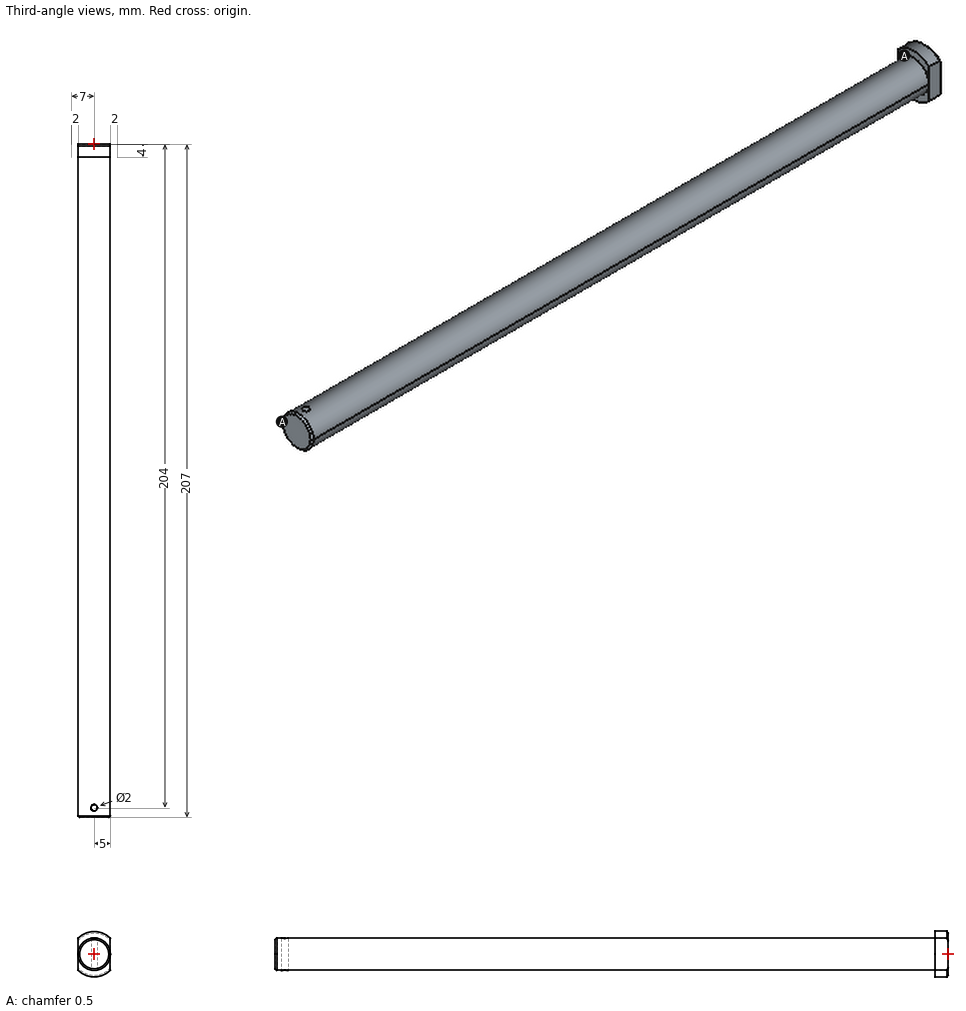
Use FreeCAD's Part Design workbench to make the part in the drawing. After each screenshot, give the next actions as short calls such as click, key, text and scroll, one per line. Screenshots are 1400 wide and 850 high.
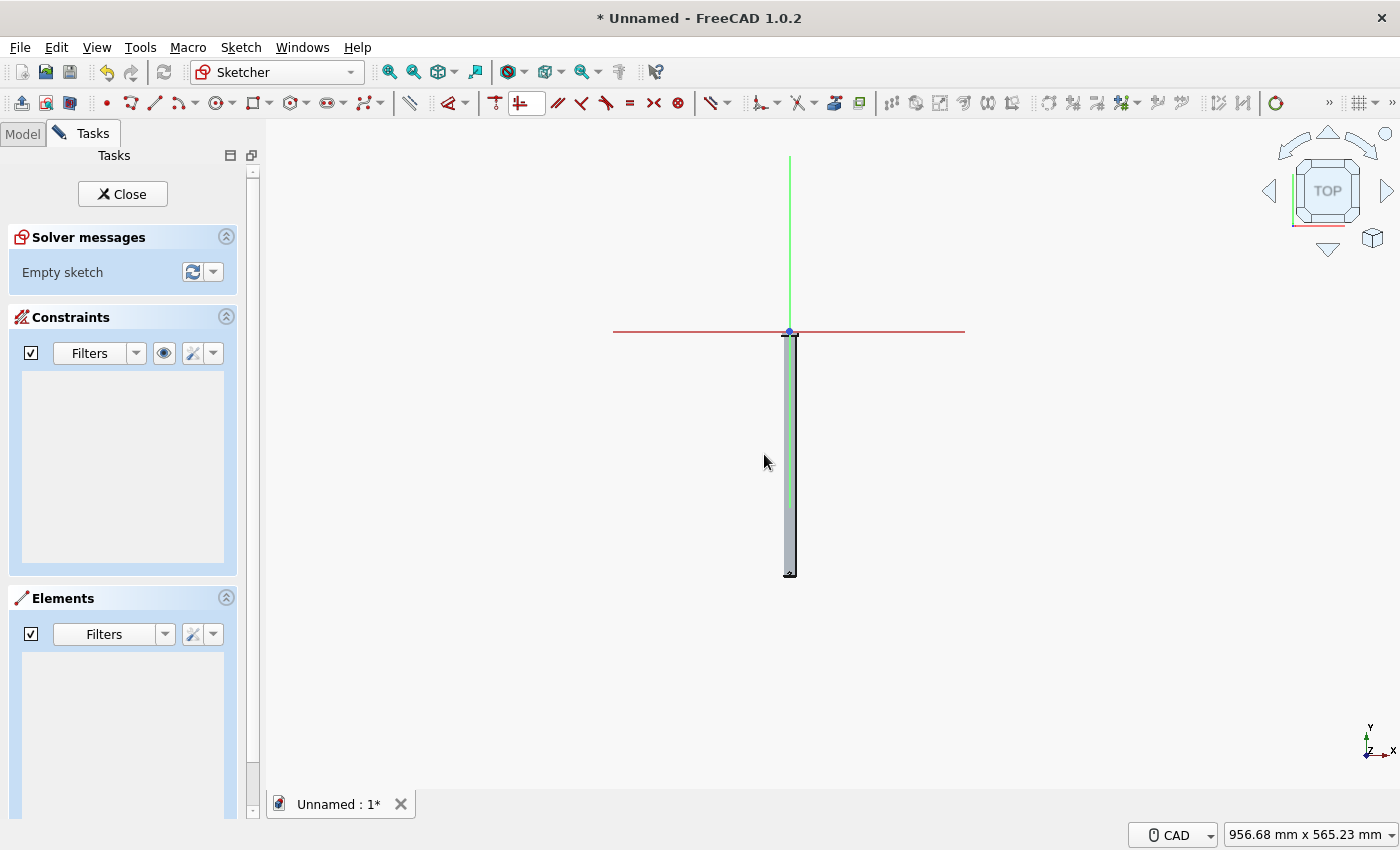
scroll(787, 328, up, 15)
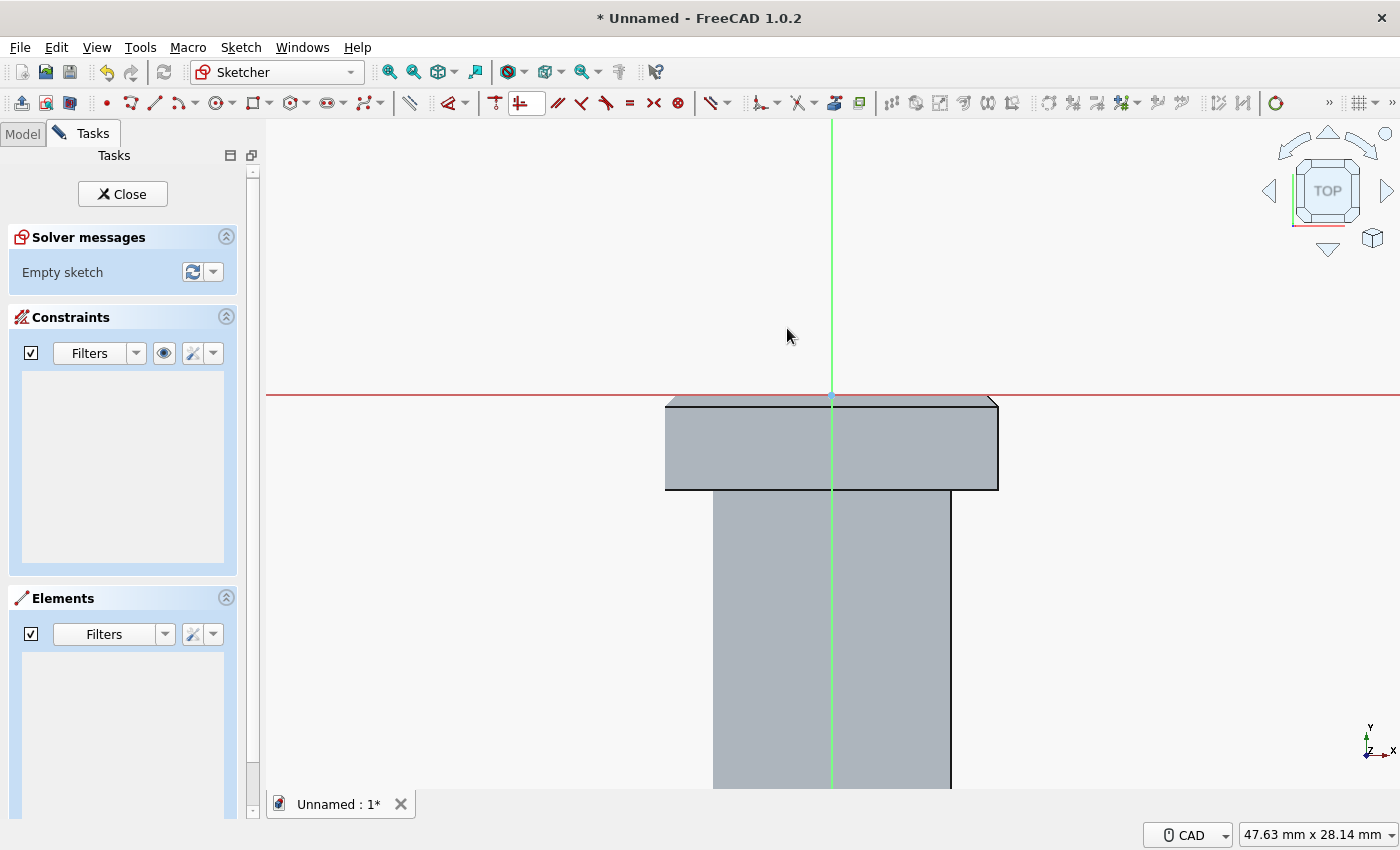
scroll(743, 439, up, 7)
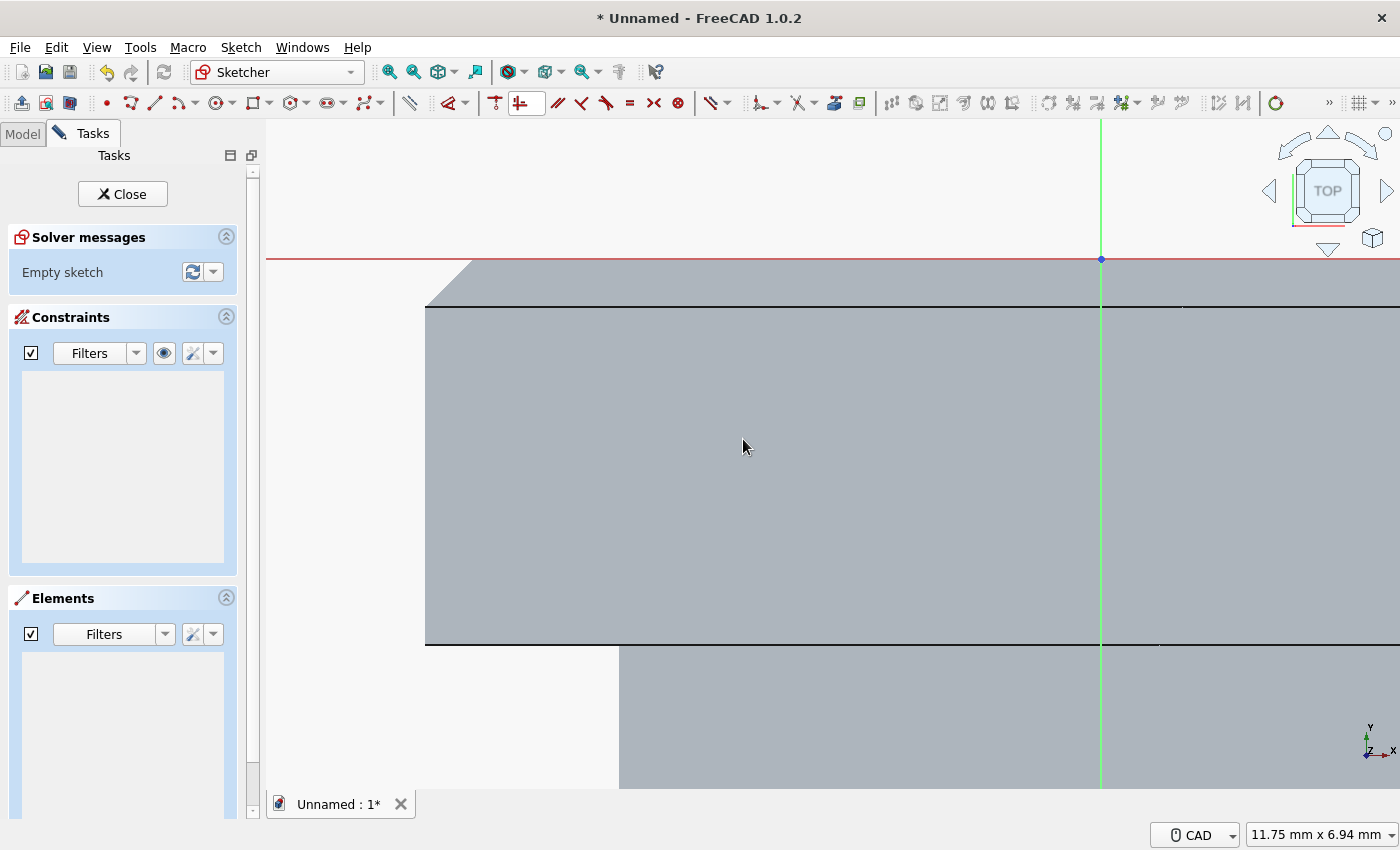
click(254, 104)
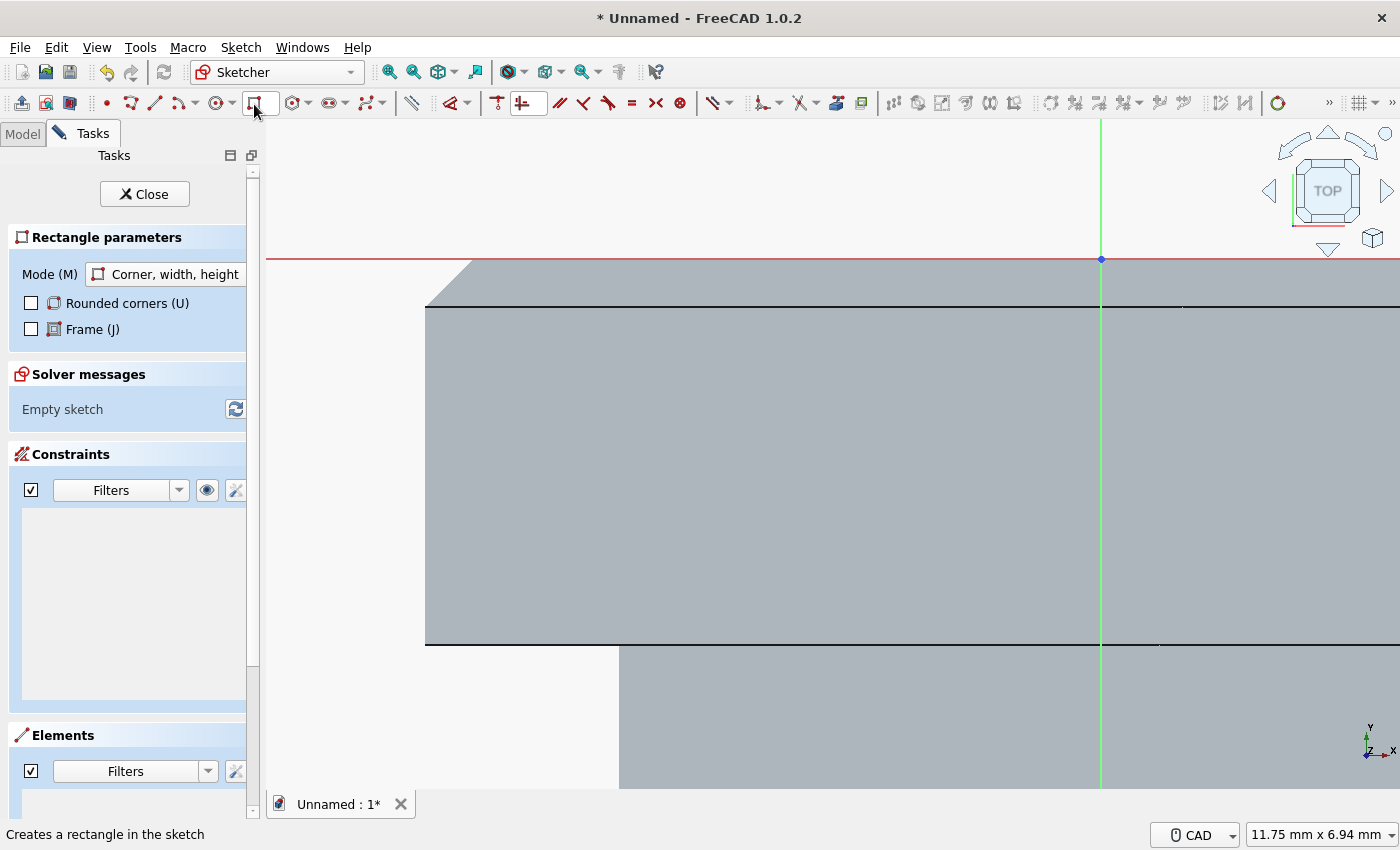
click(426, 259)
click(619, 645)
key(Escape)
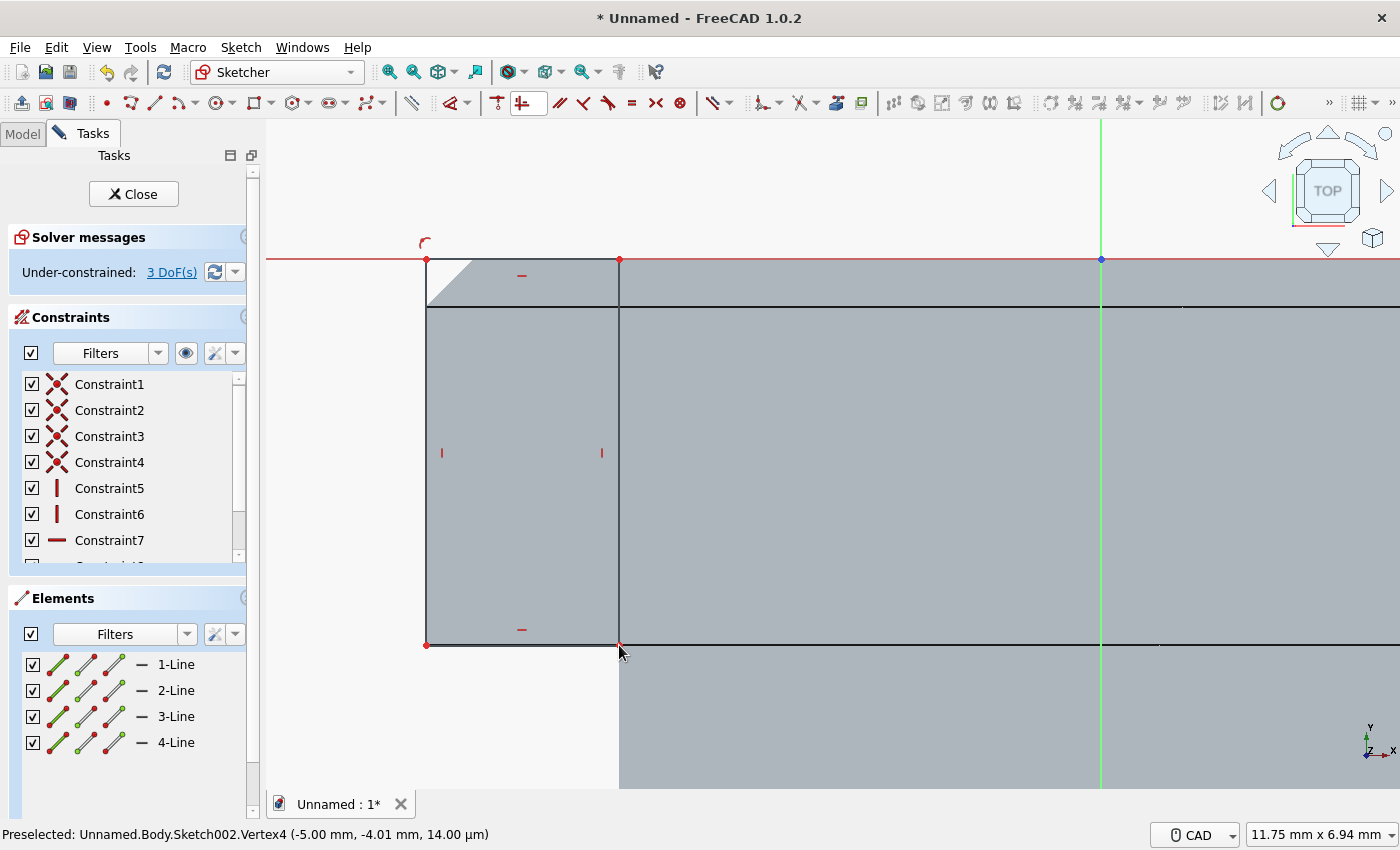
click(450, 104)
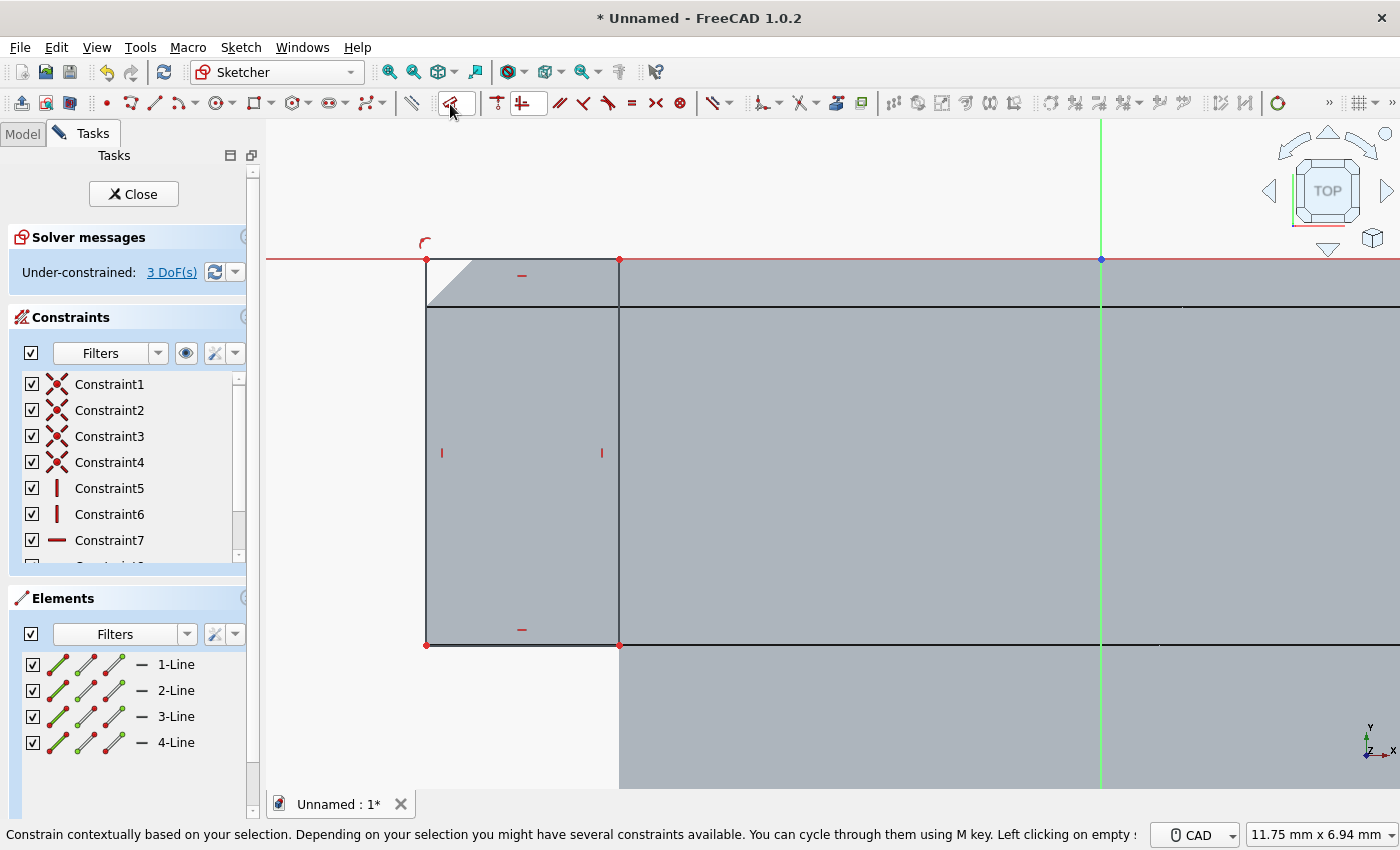
click(426, 375)
click(392, 453)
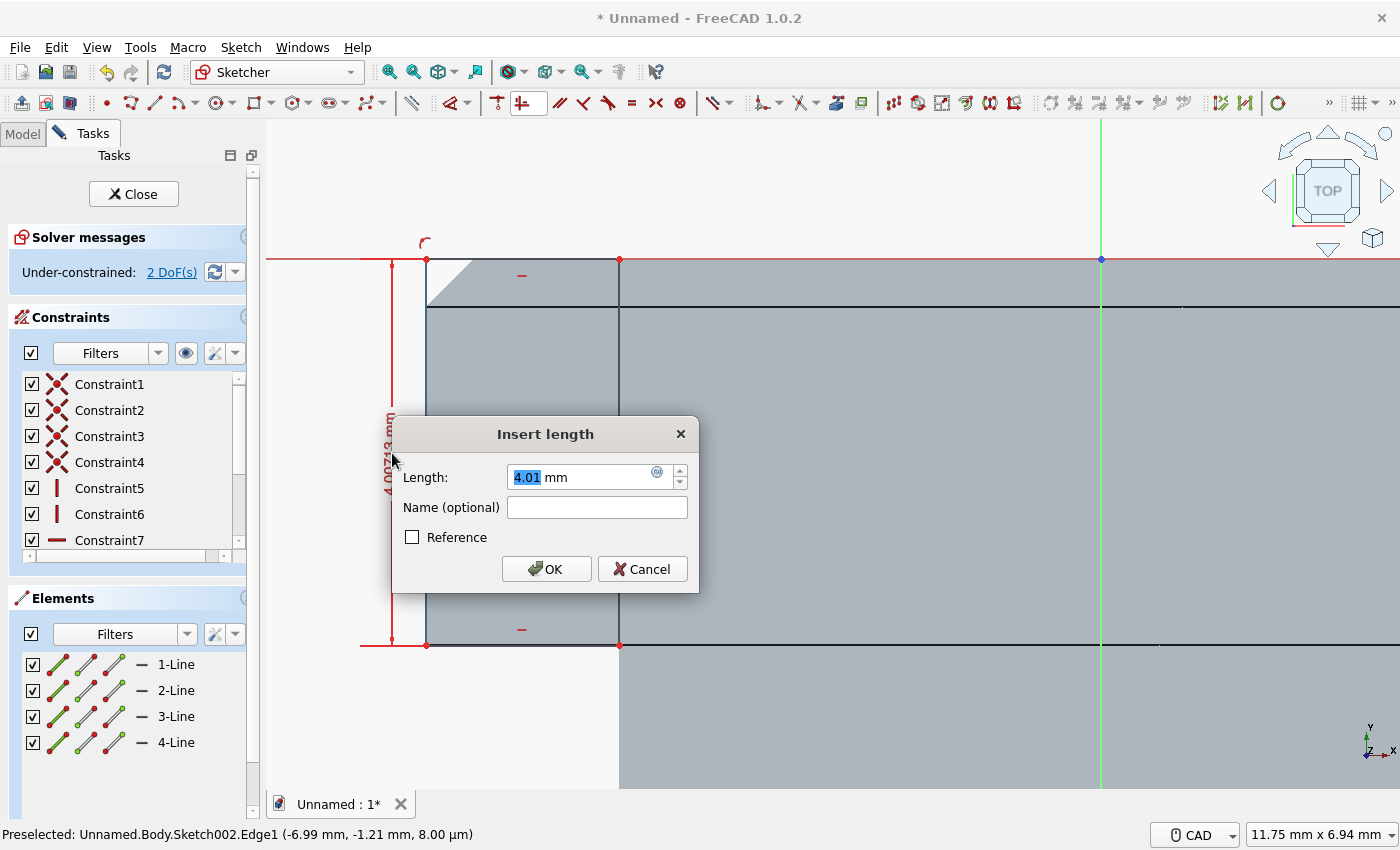
text(4)
key(Return)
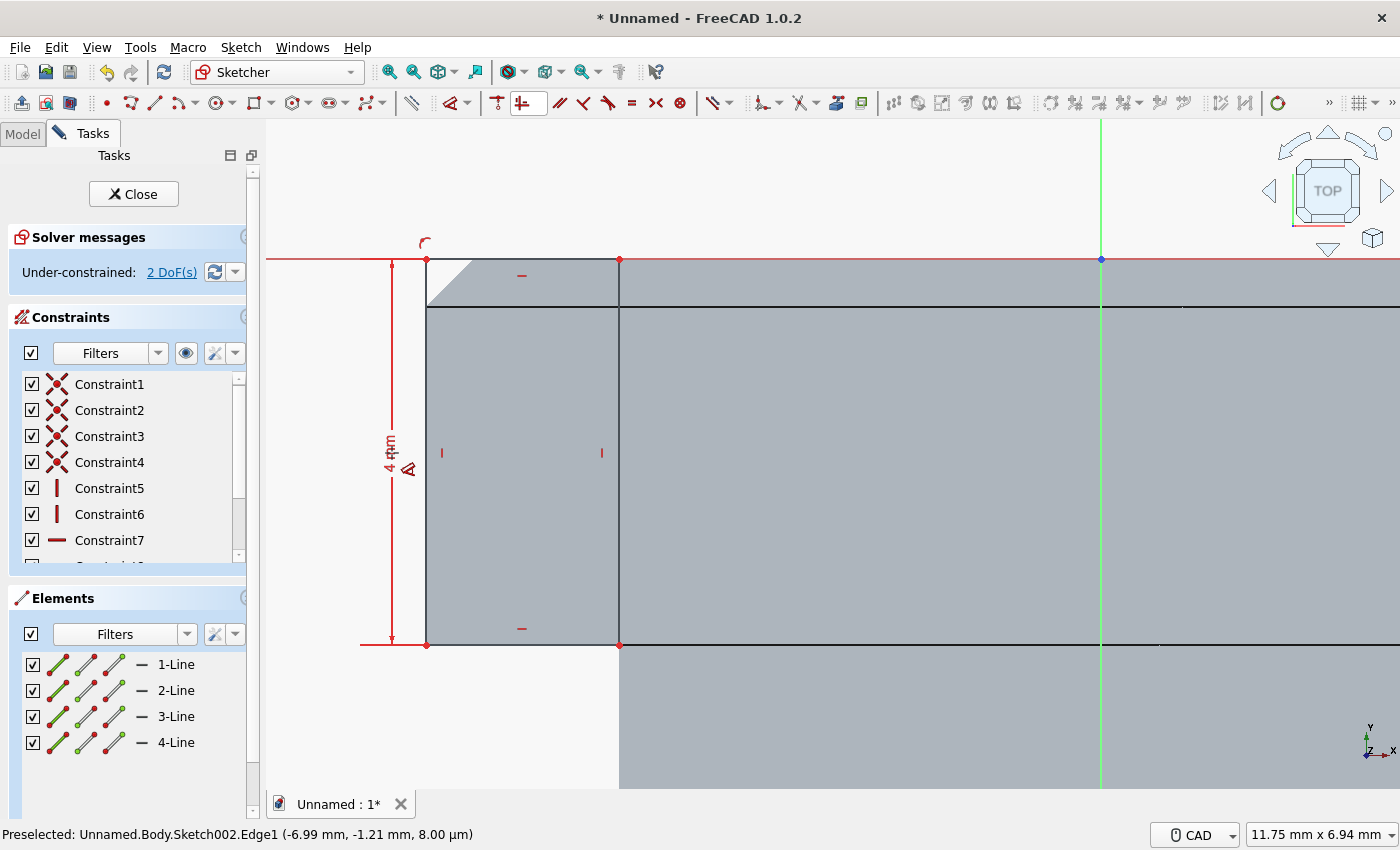
click(484, 645)
click(522, 679)